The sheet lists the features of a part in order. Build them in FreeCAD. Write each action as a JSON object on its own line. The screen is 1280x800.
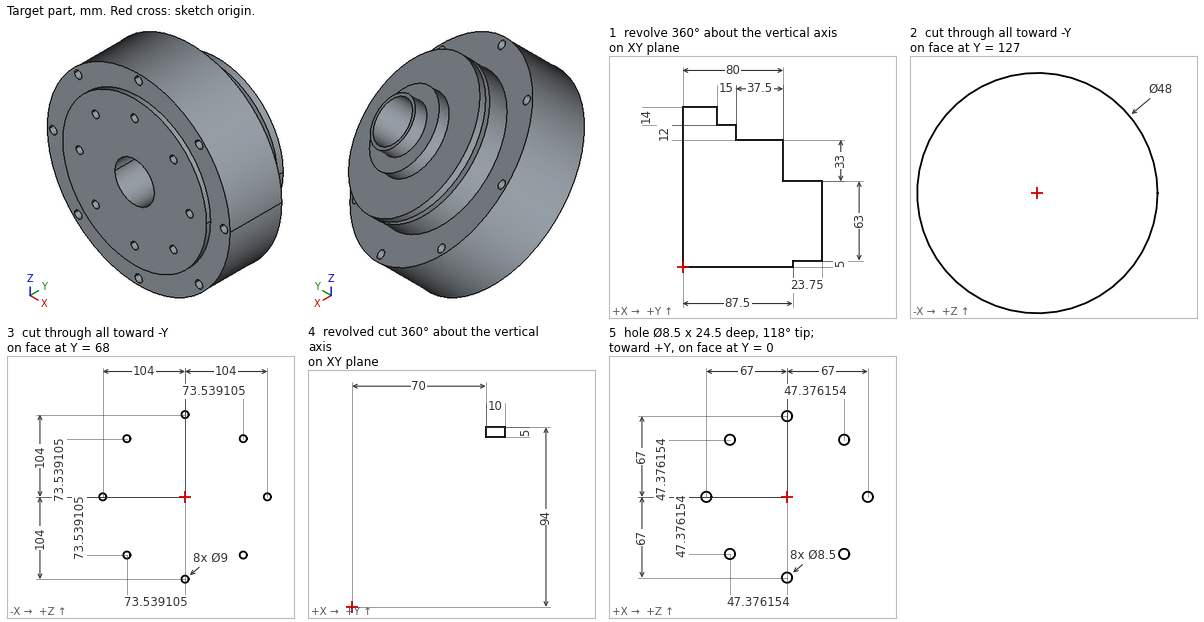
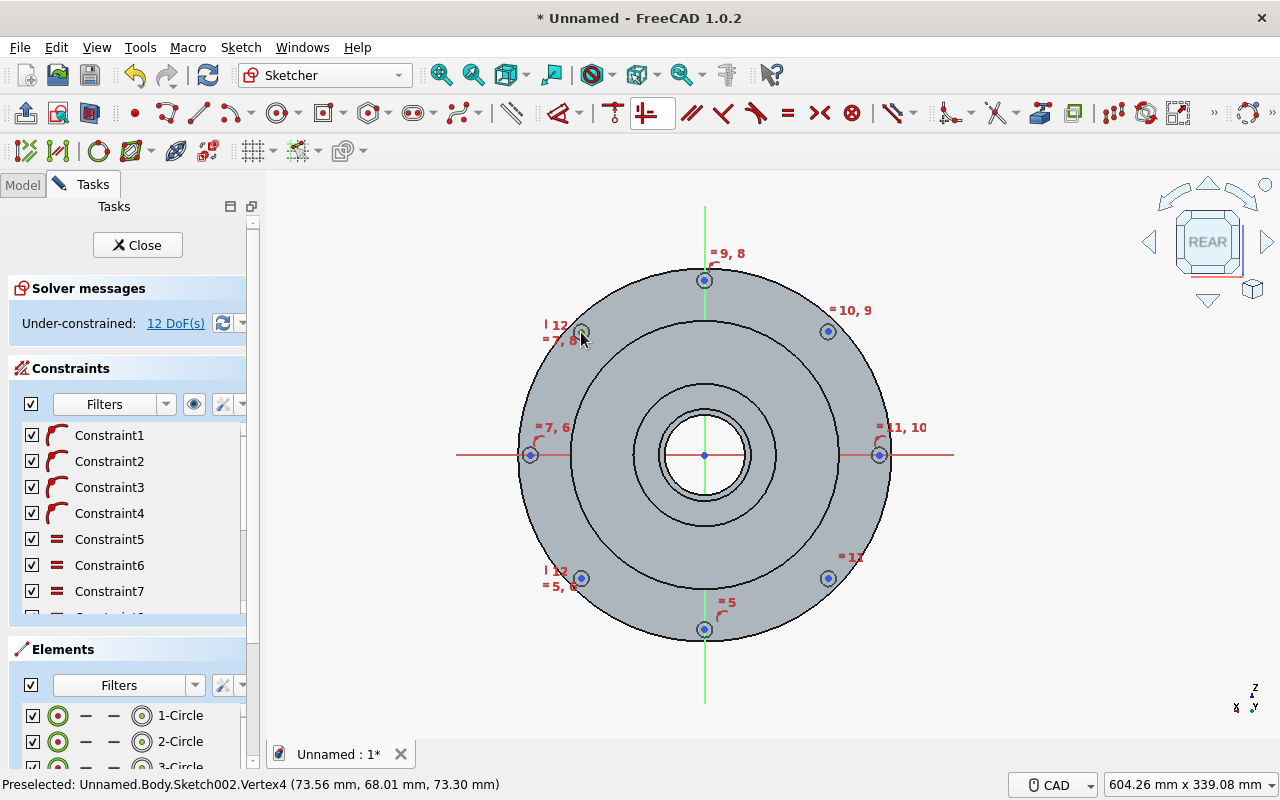
{"action": "left_click", "coordinate": [828, 332]}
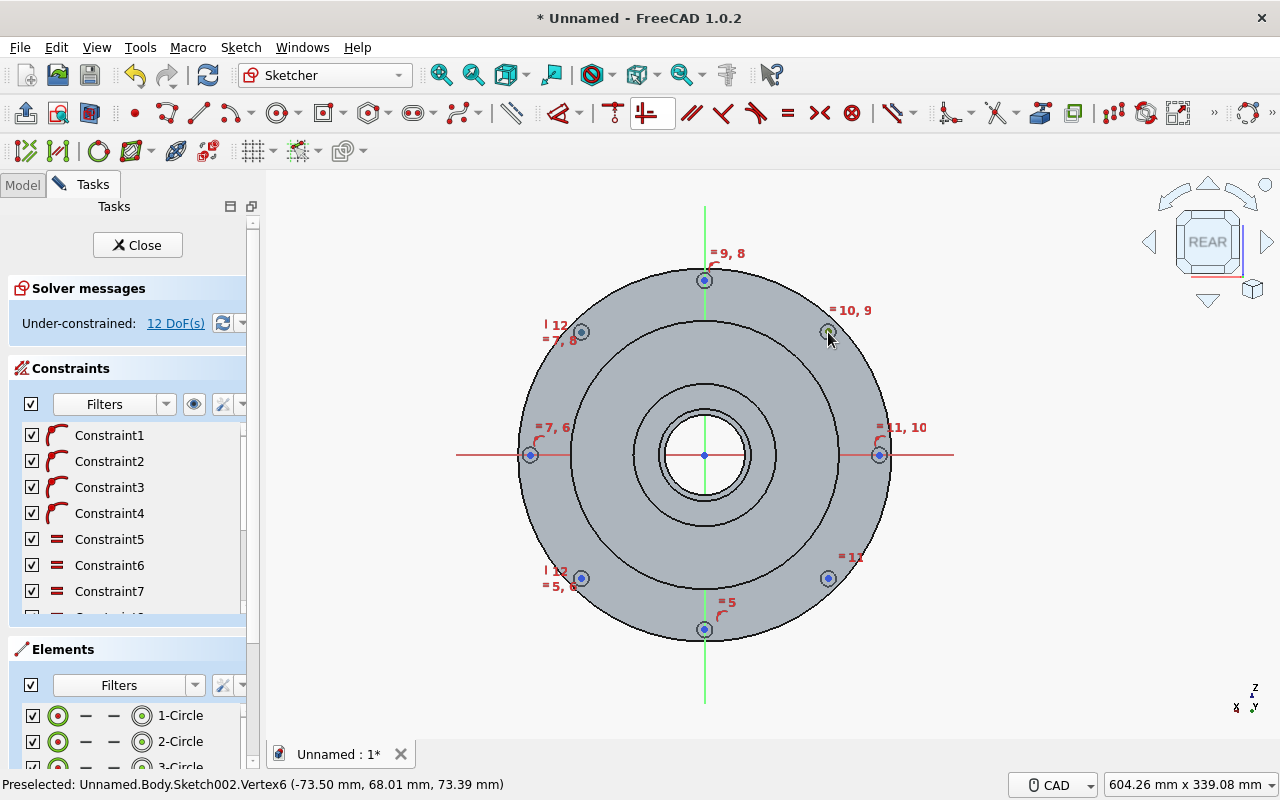
{"action": "key", "text": "h"}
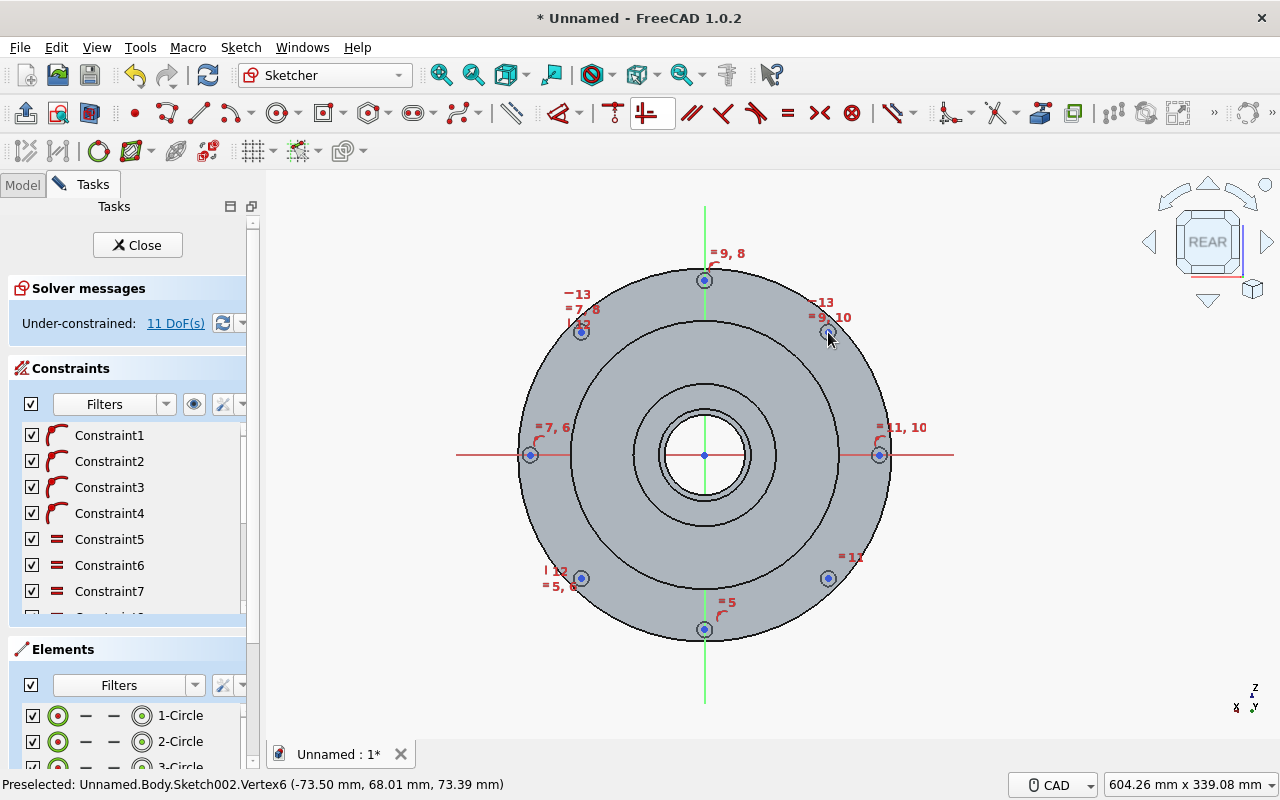
{"action": "left_click", "coordinate": [828, 332]}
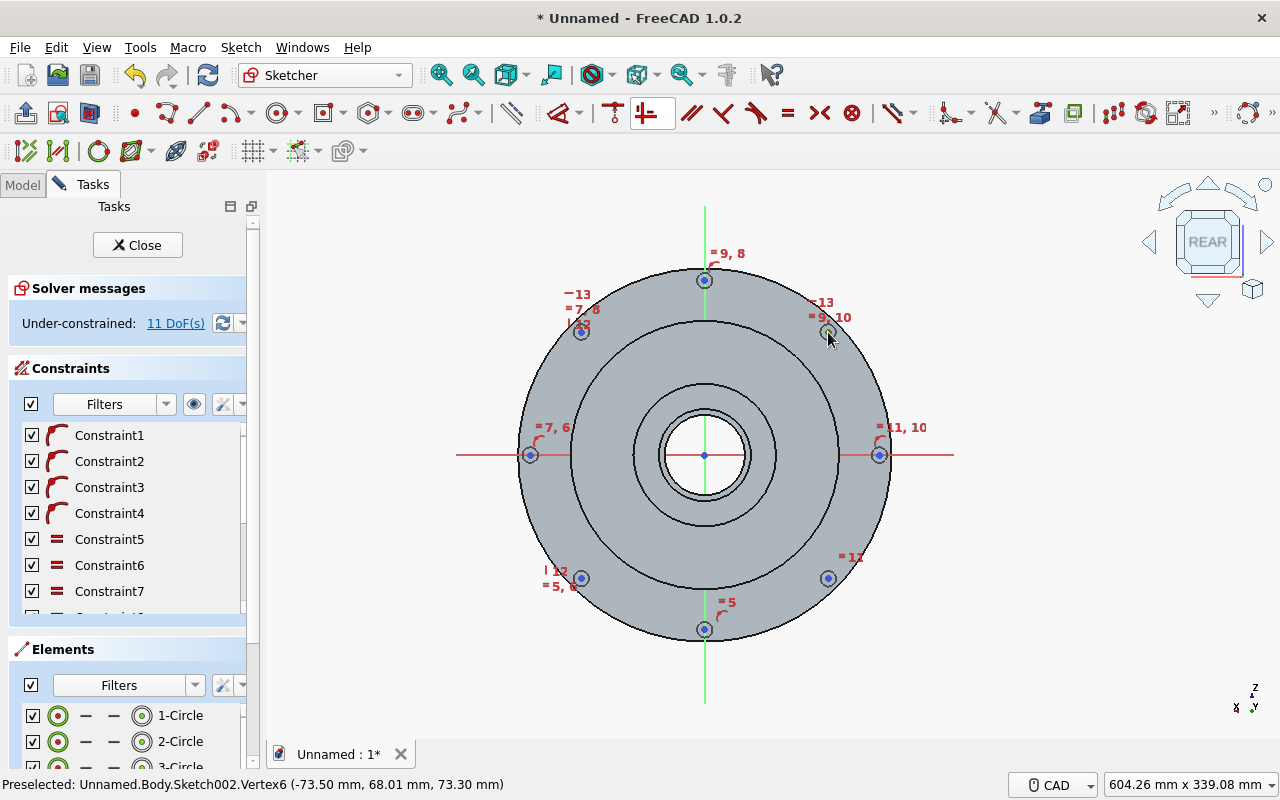
{"action": "left_click", "coordinate": [828, 579]}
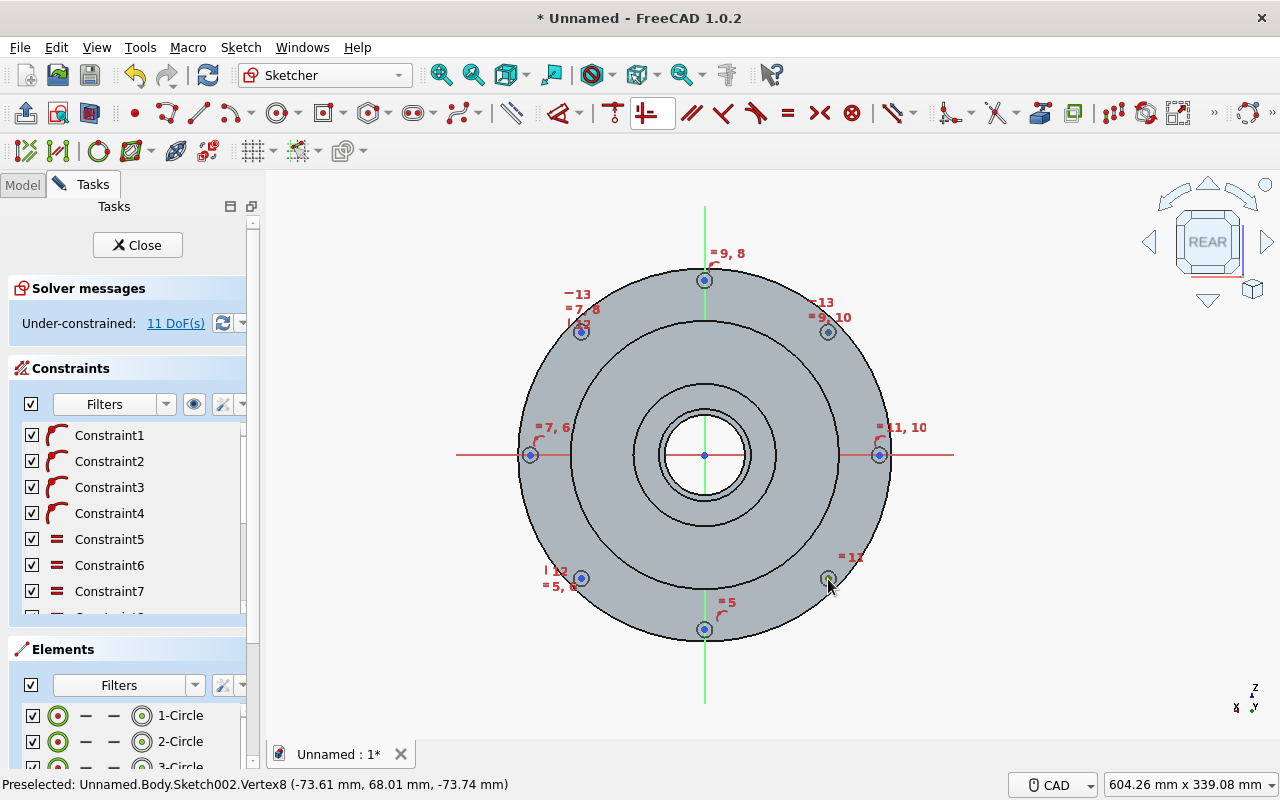
{"action": "left_click", "coordinate": [670, 114]}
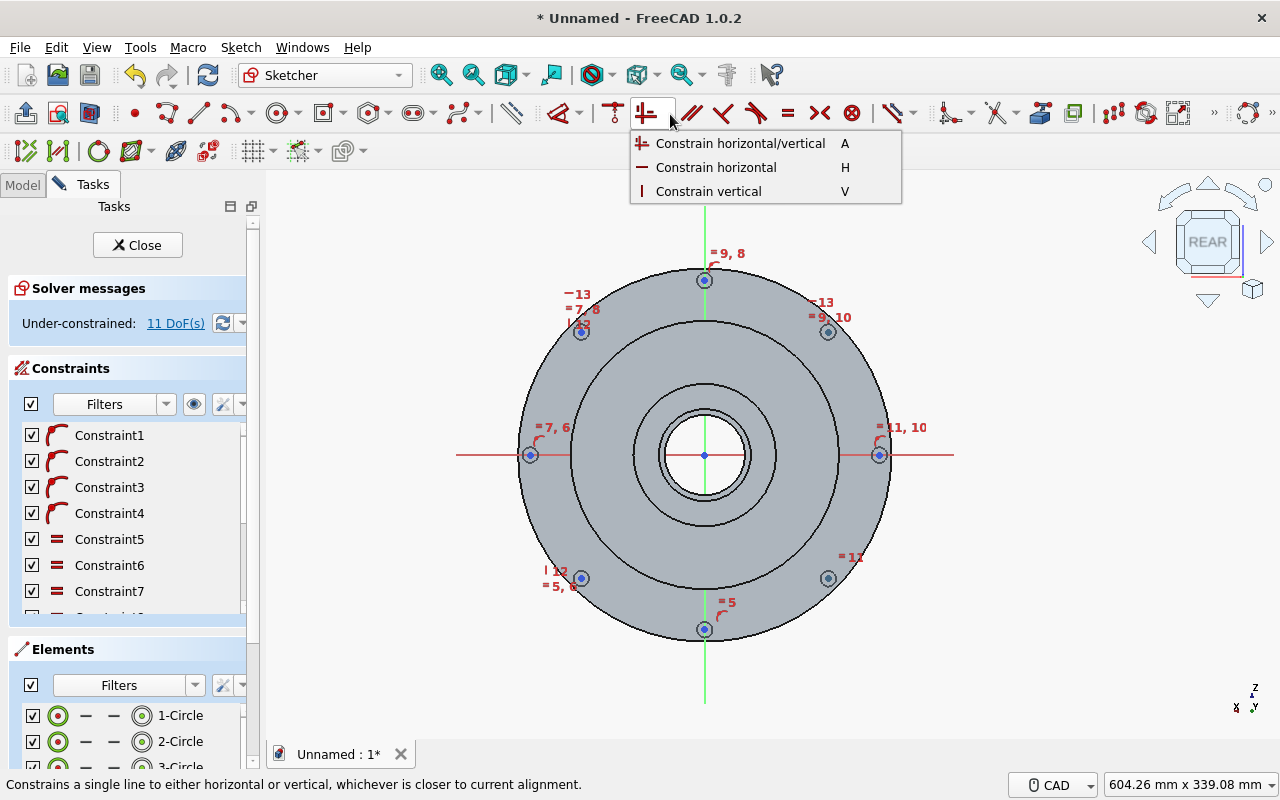
{"action": "left_click", "coordinate": [766, 191]}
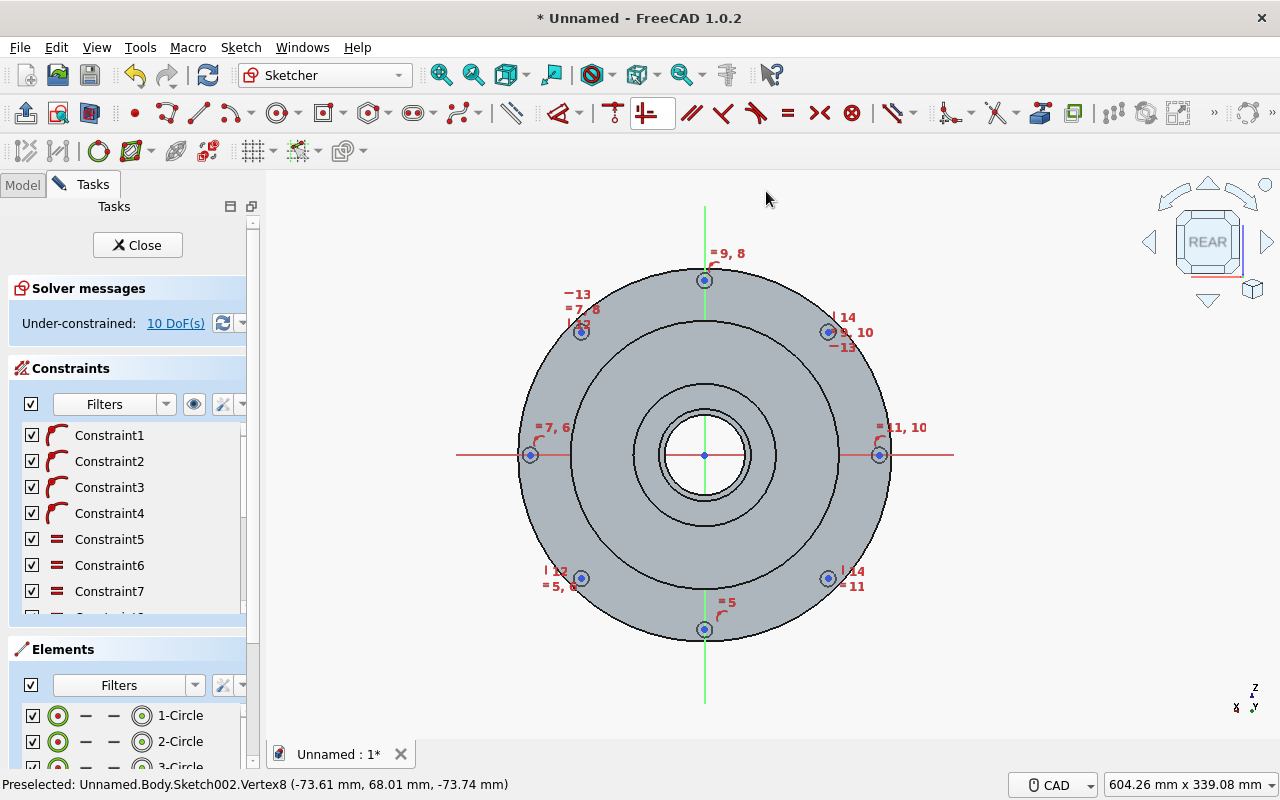
{"action": "left_click", "coordinate": [581, 579]}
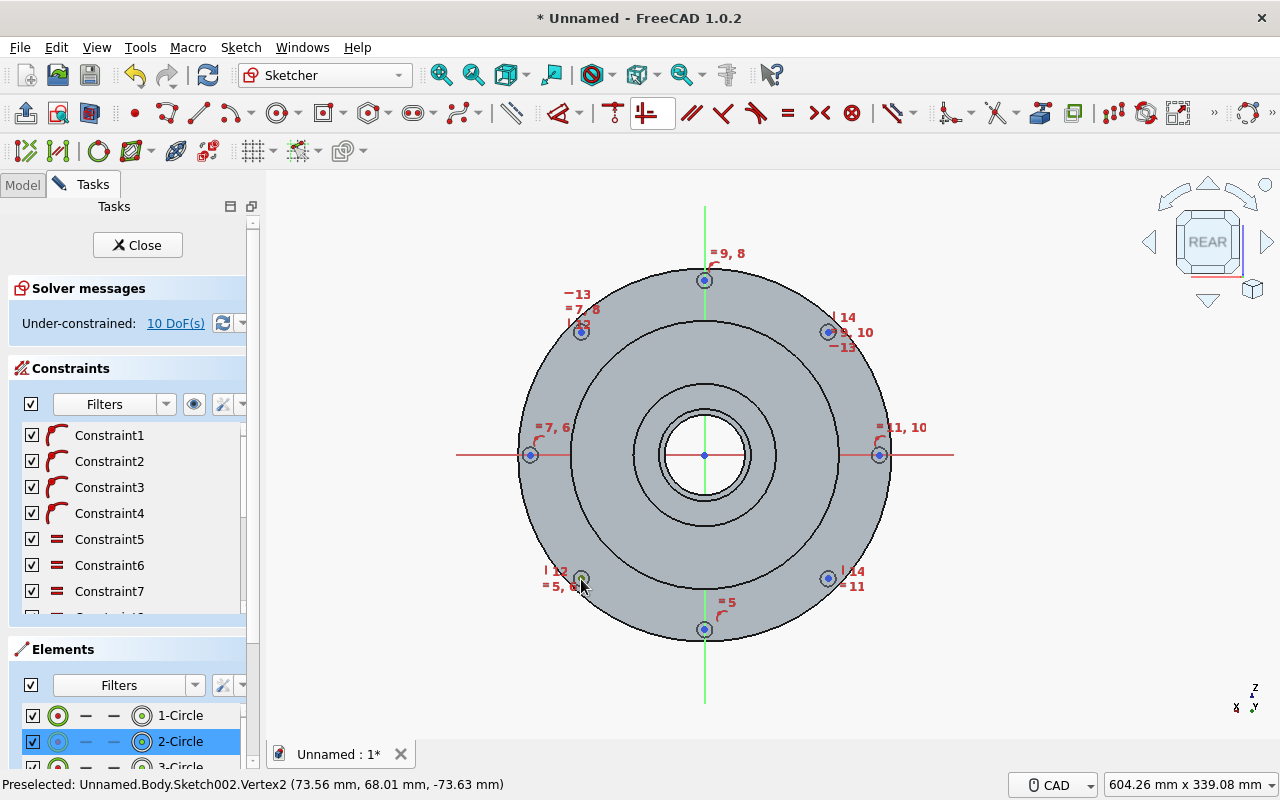
{"action": "left_click", "coordinate": [828, 579]}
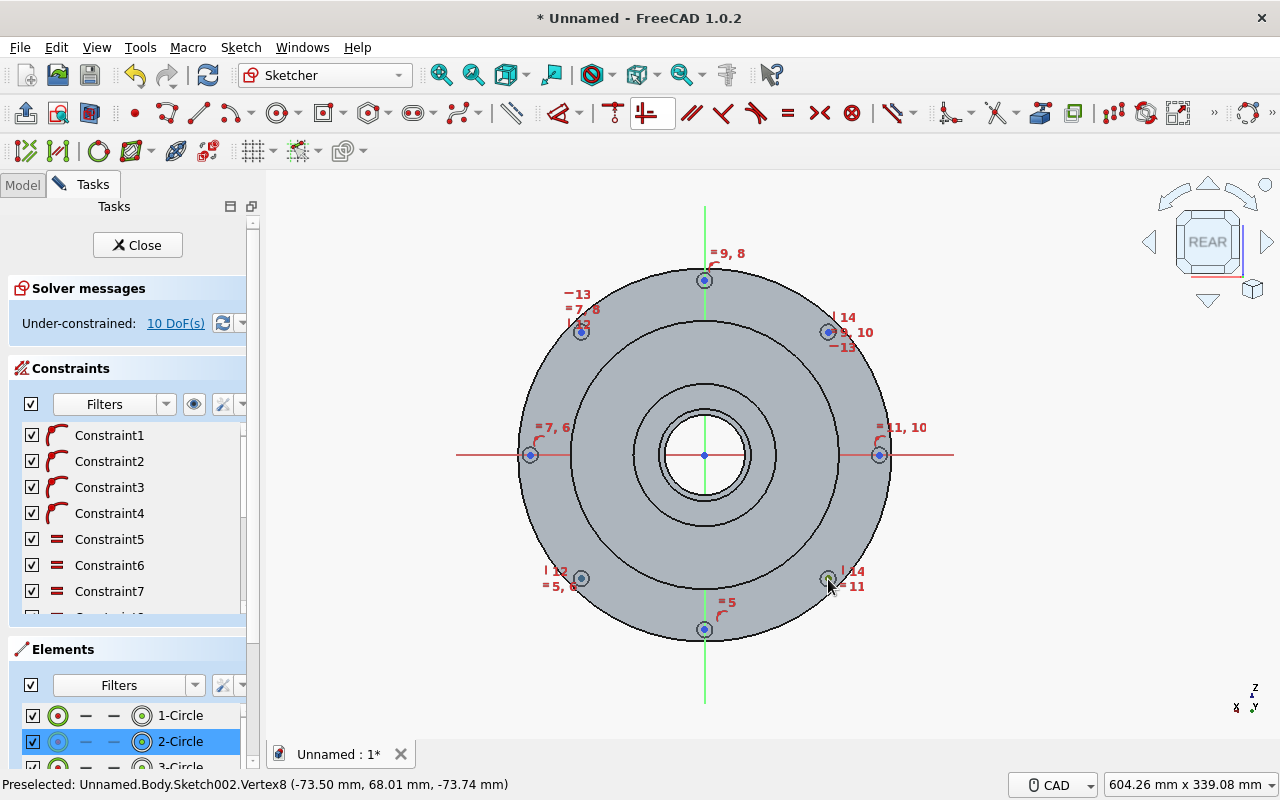
{"action": "key", "text": "h"}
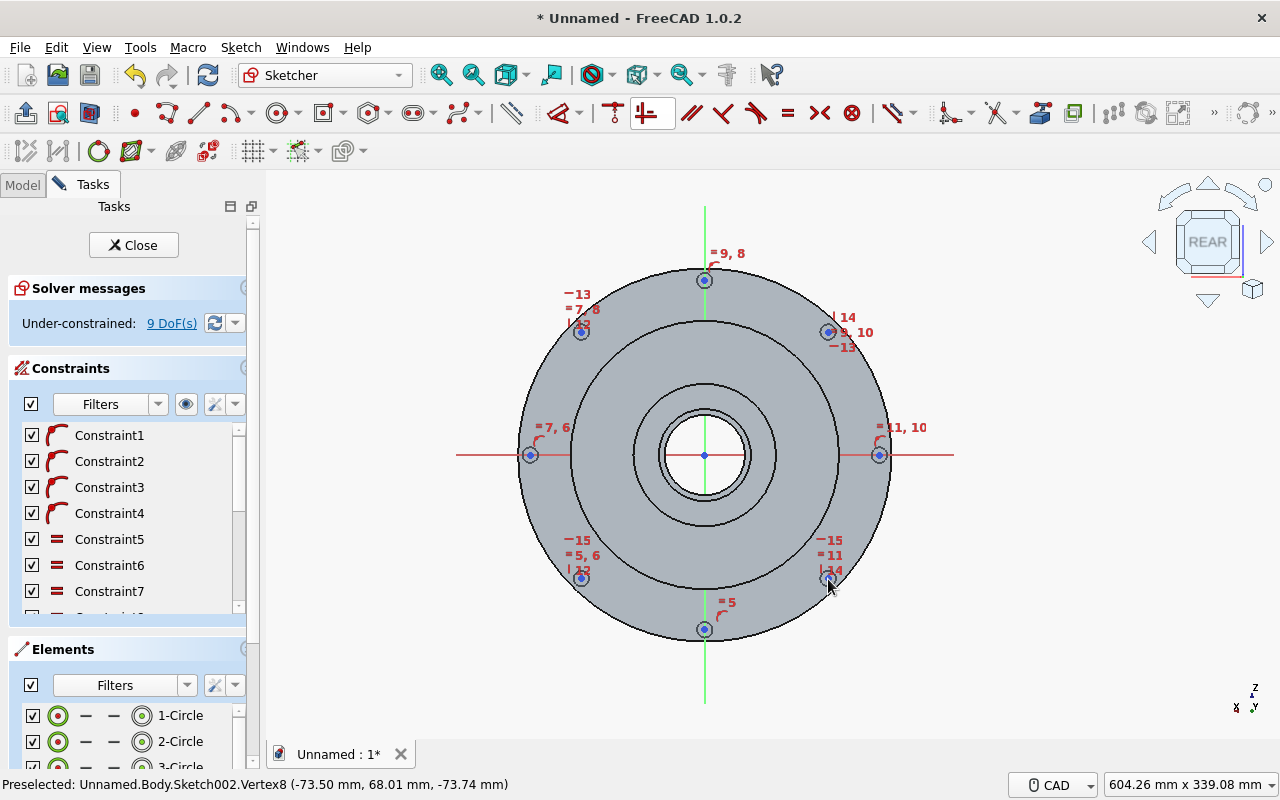
{"action": "left_click", "coordinate": [558, 114]}